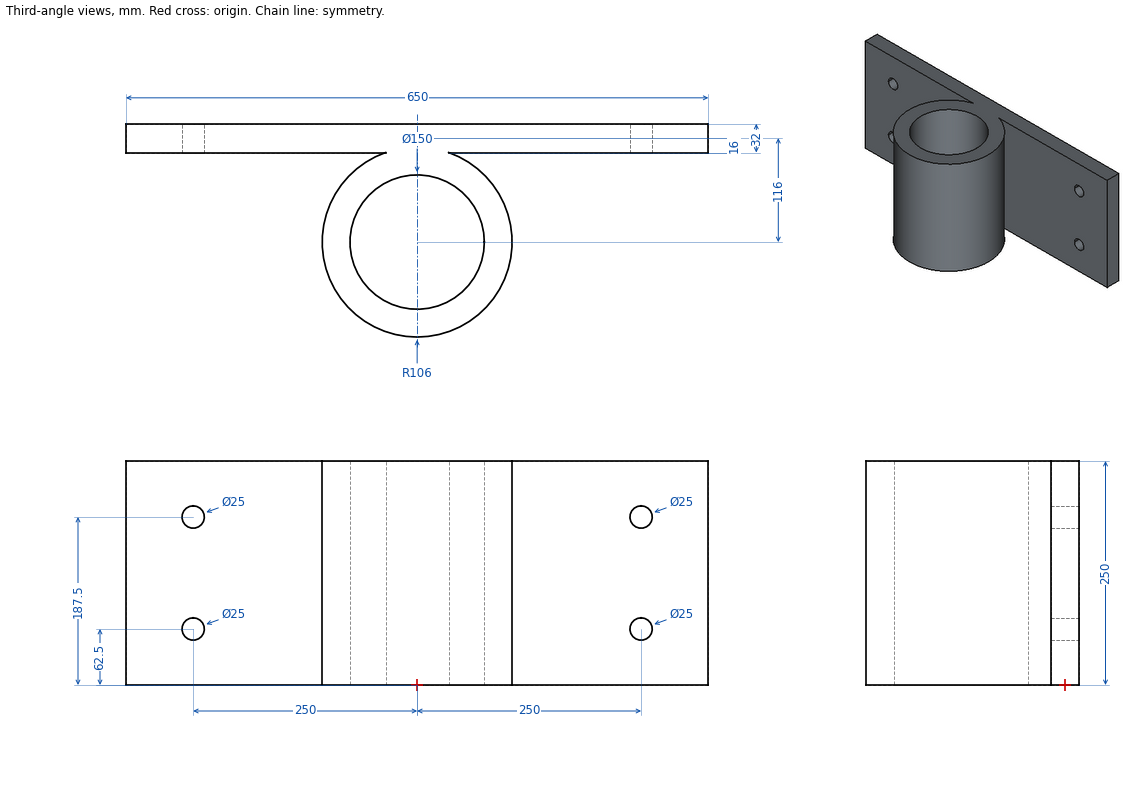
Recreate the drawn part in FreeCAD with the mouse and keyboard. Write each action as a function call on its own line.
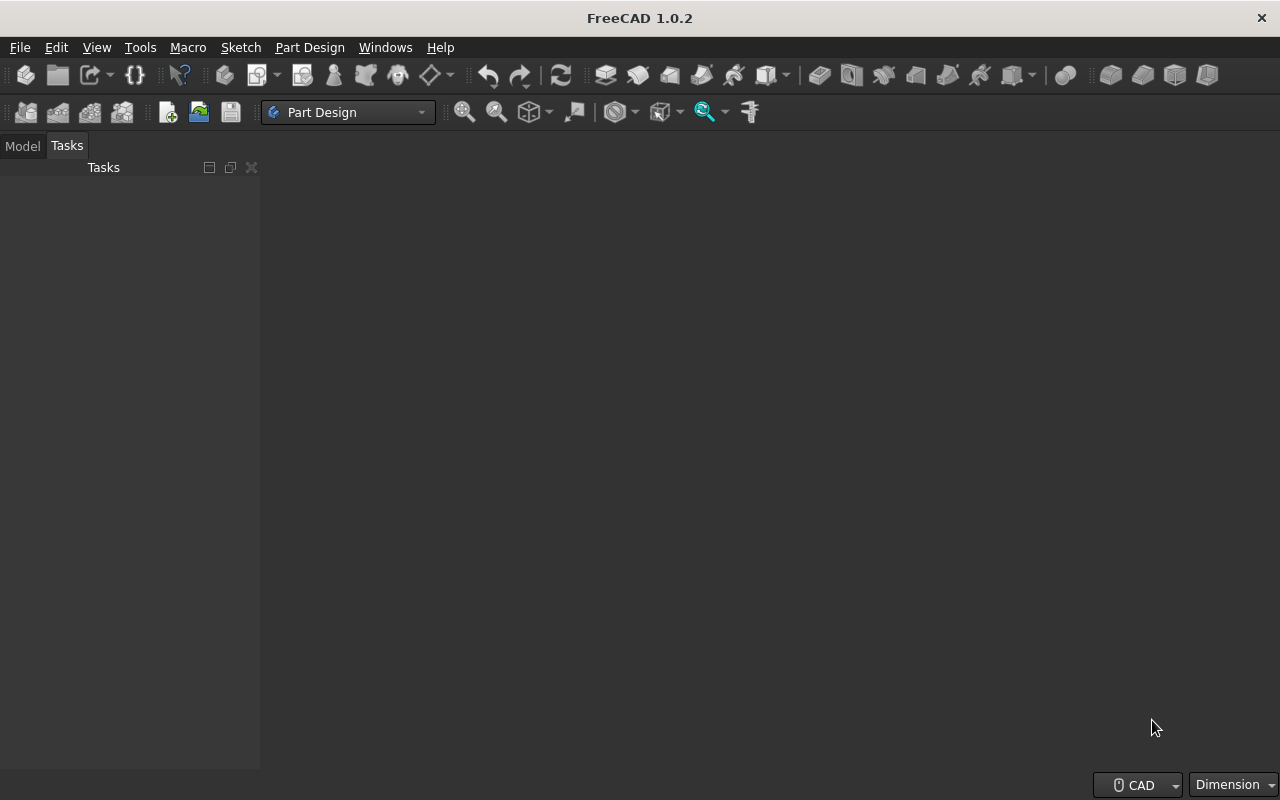
click(168, 112)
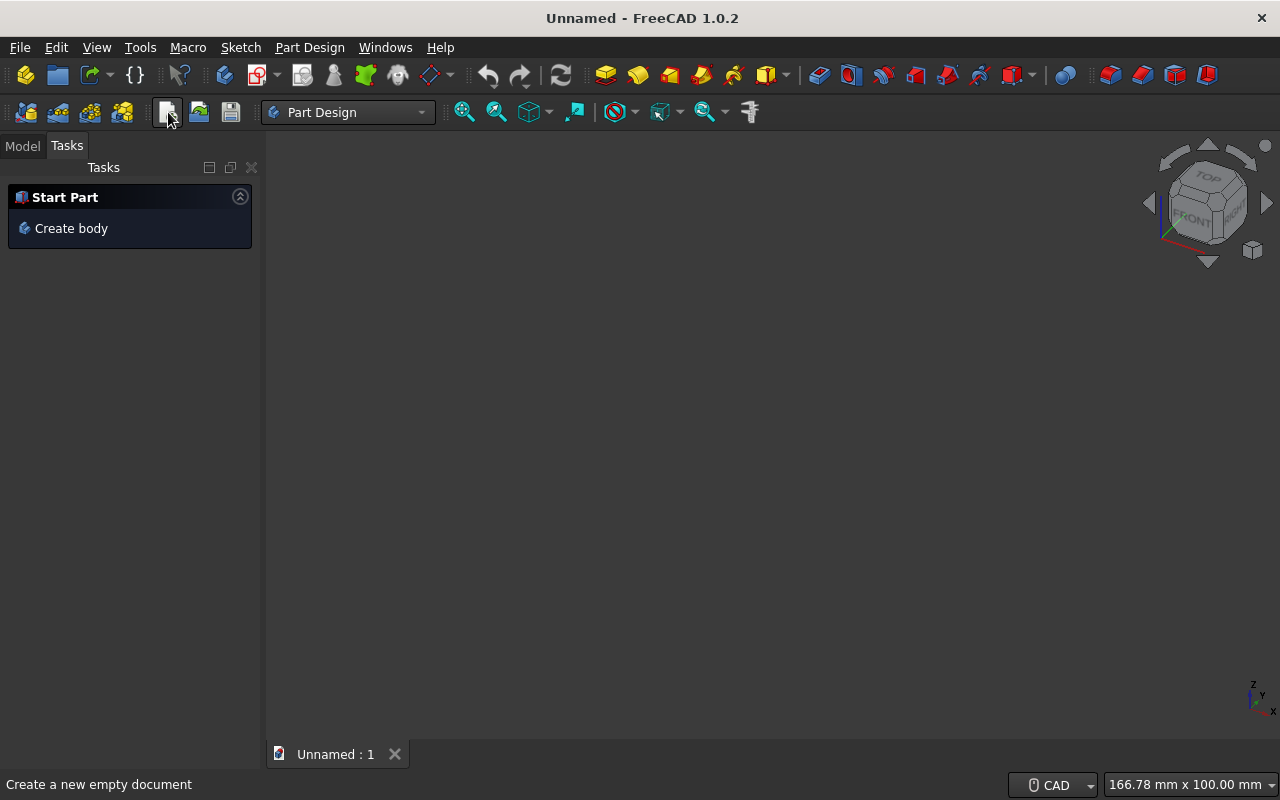
click(258, 76)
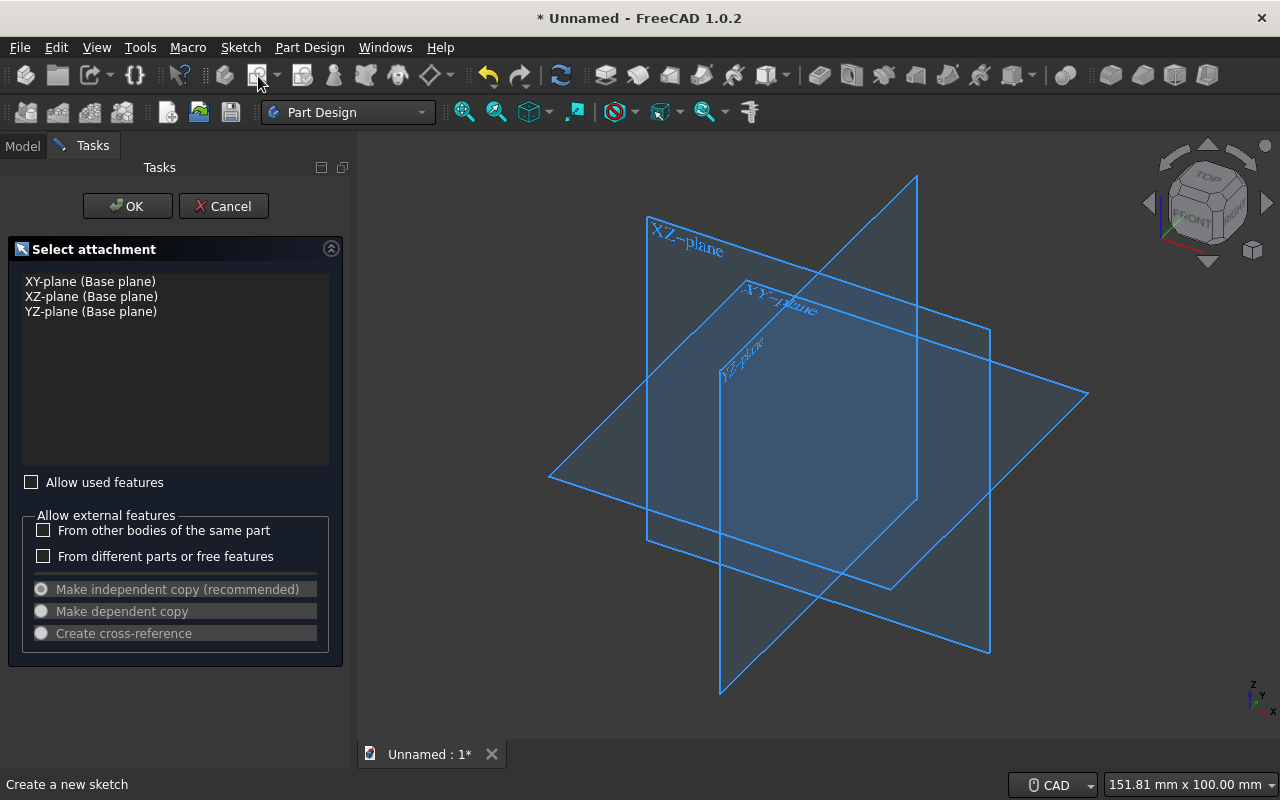
click(82, 282)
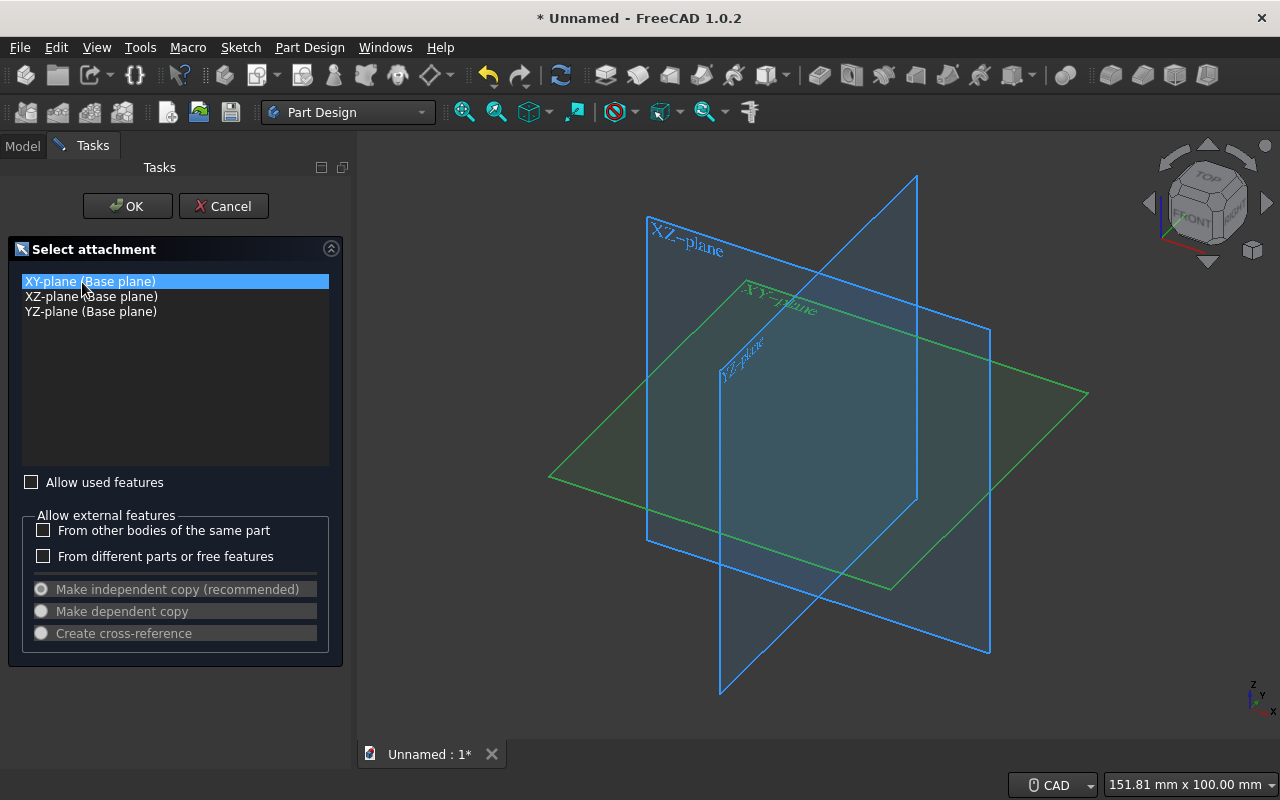
click(128, 206)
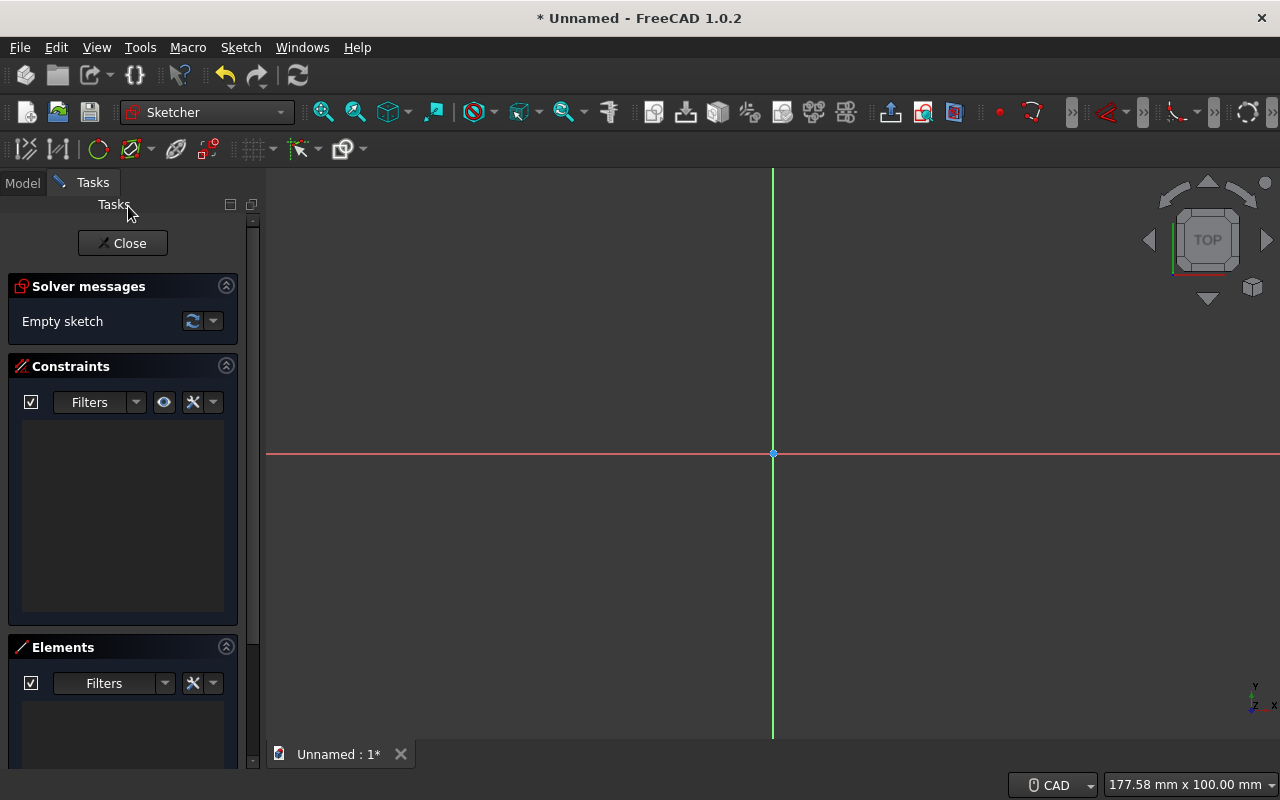
scroll(691, 337, down, 9)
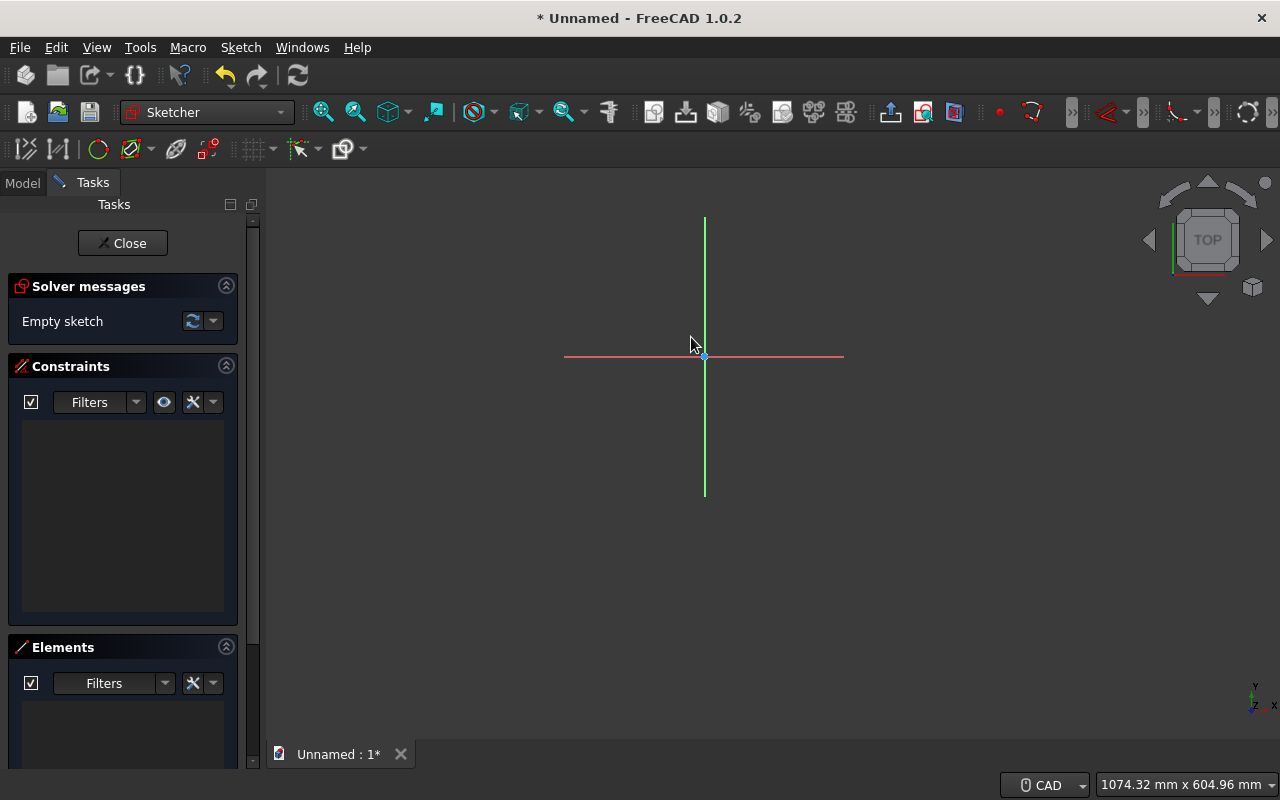
click(1032, 112)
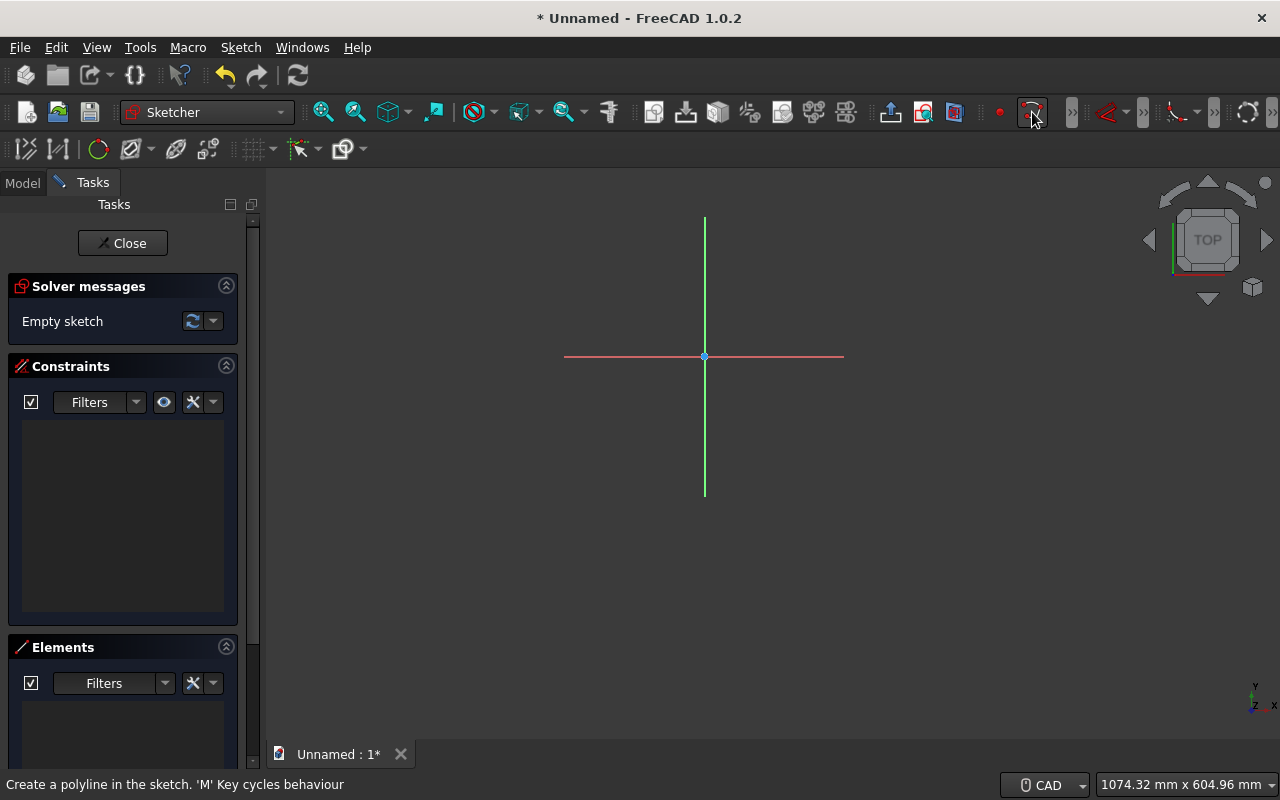
click(738, 372)
click(1012, 372)
click(1012, 341)
click(398, 341)
click(398, 372)
click(672, 372)
right_click(672, 372)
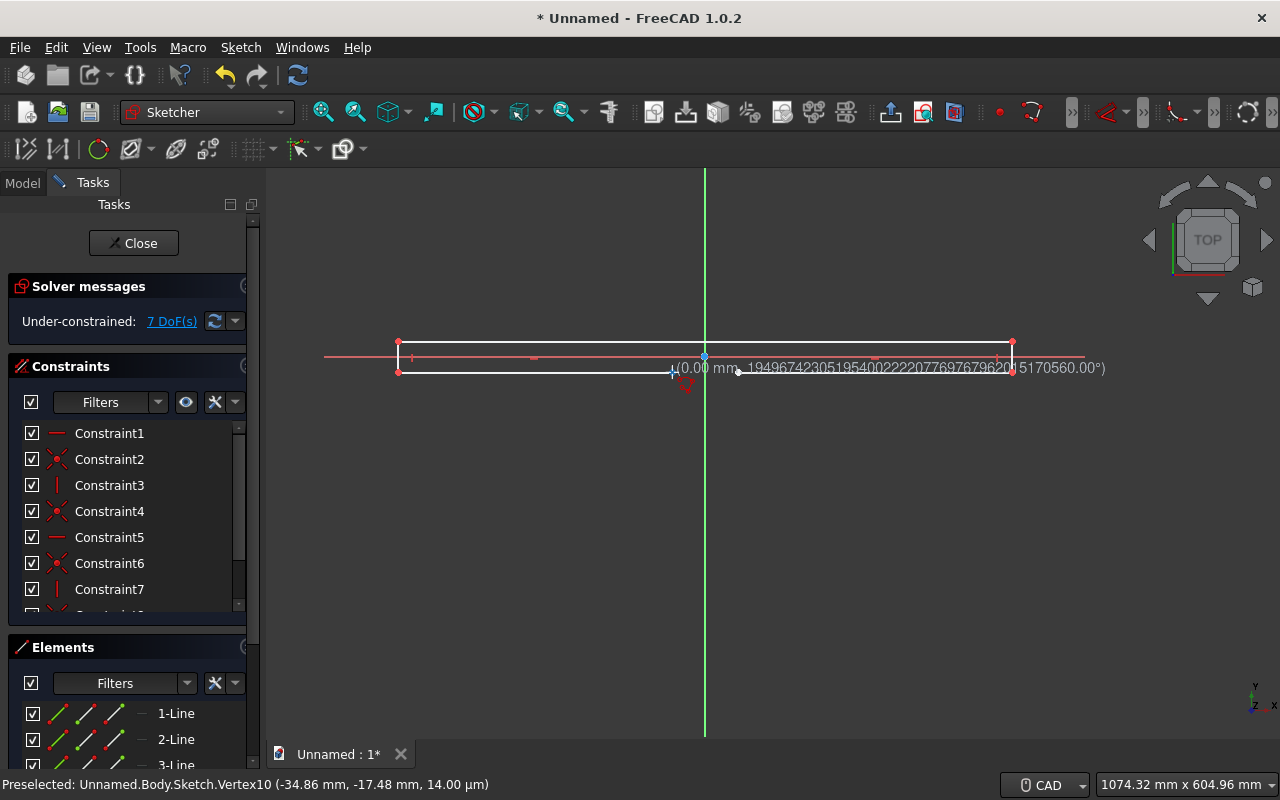
key(g)
key(3)
key(a)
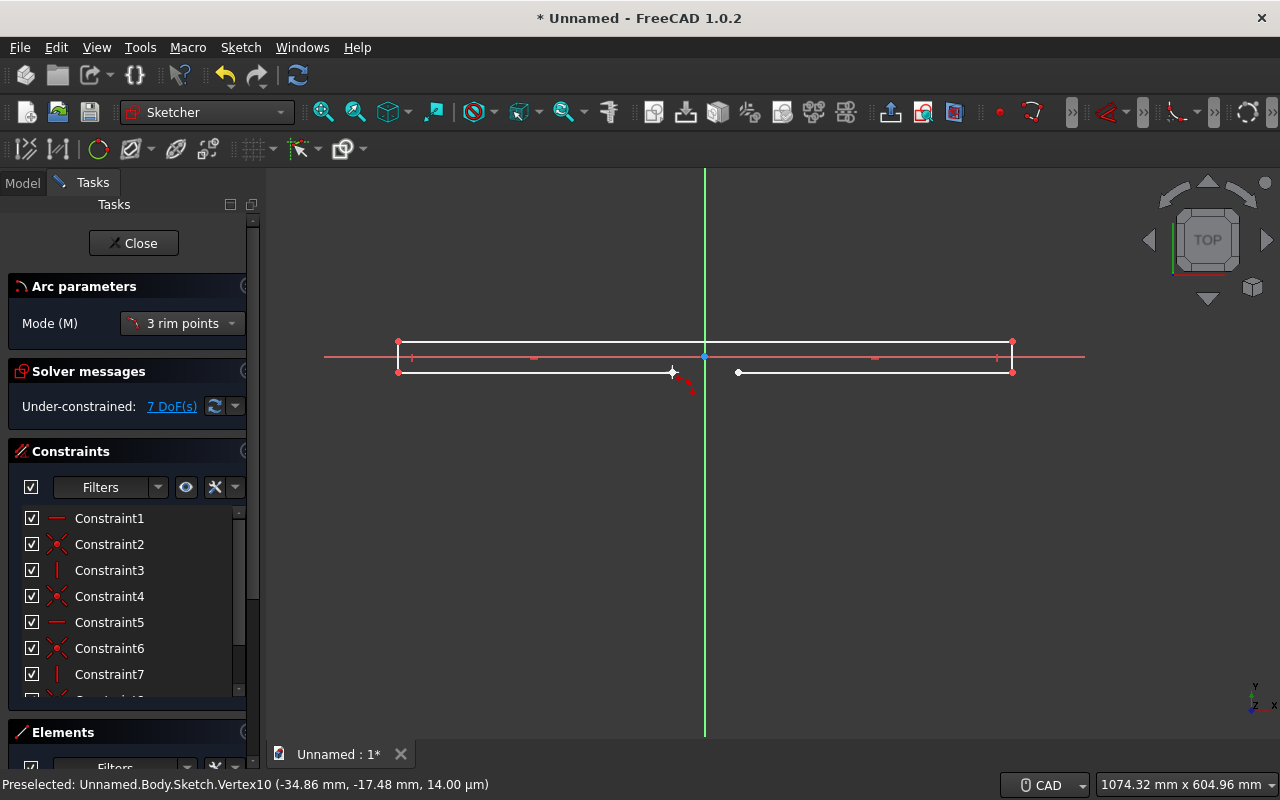
click(672, 373)
click(738, 373)
click(652, 551)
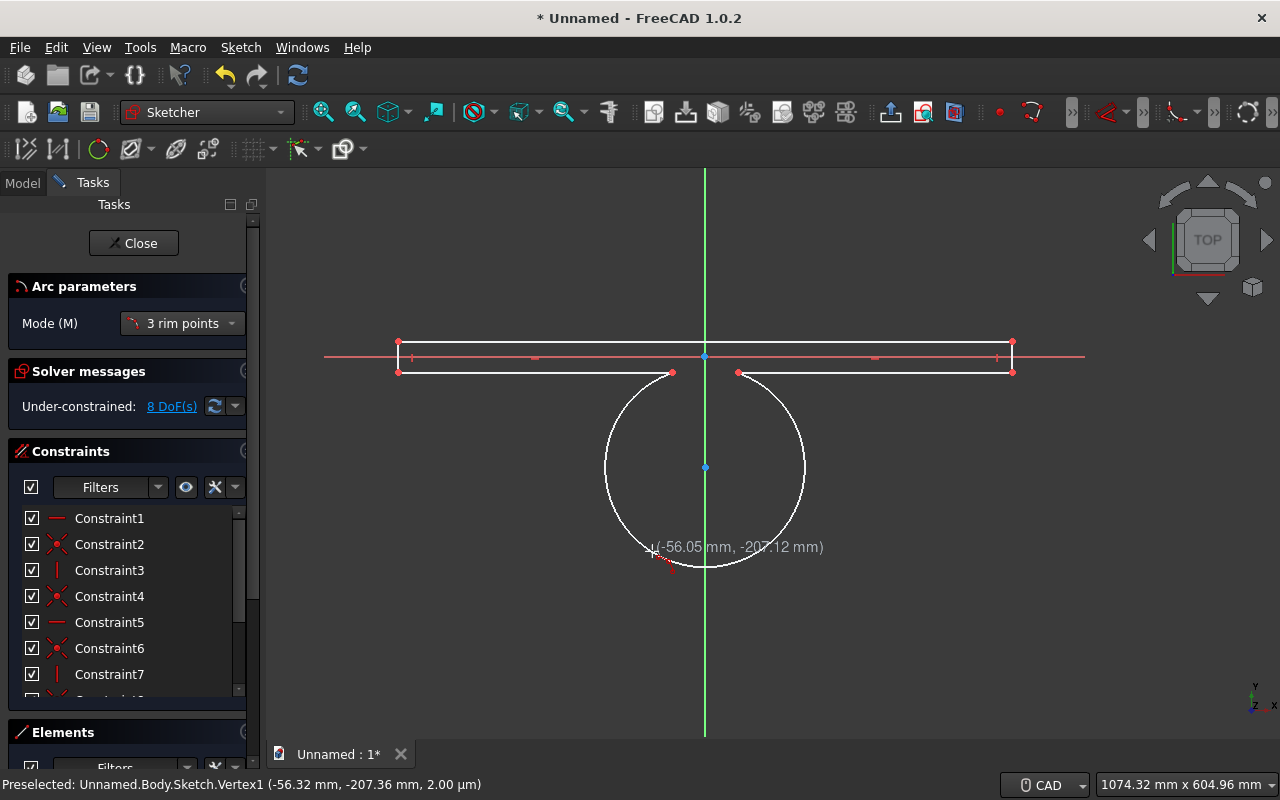
key(g)
key(c)